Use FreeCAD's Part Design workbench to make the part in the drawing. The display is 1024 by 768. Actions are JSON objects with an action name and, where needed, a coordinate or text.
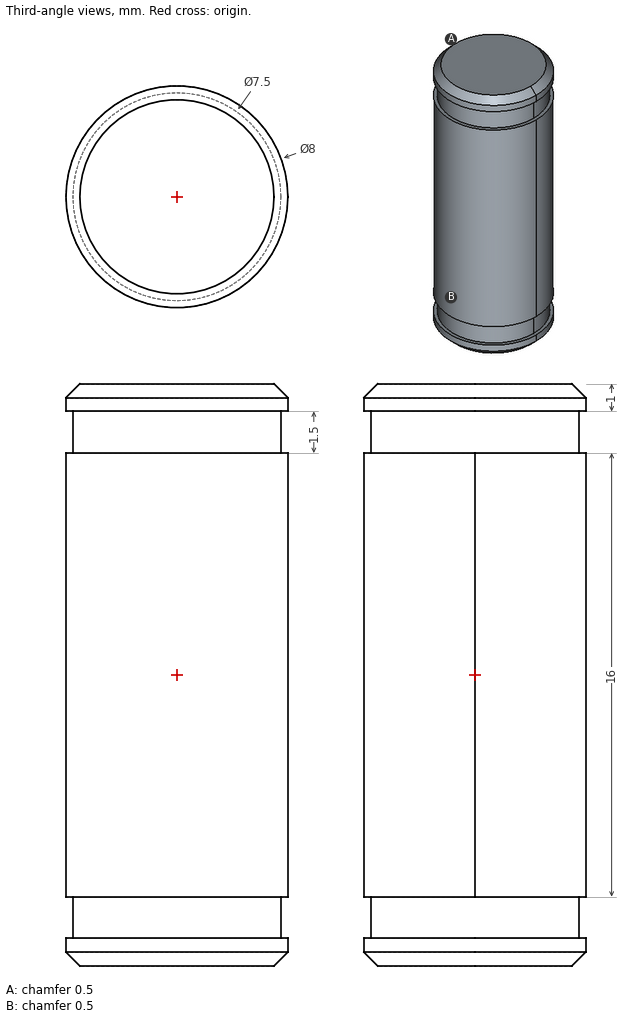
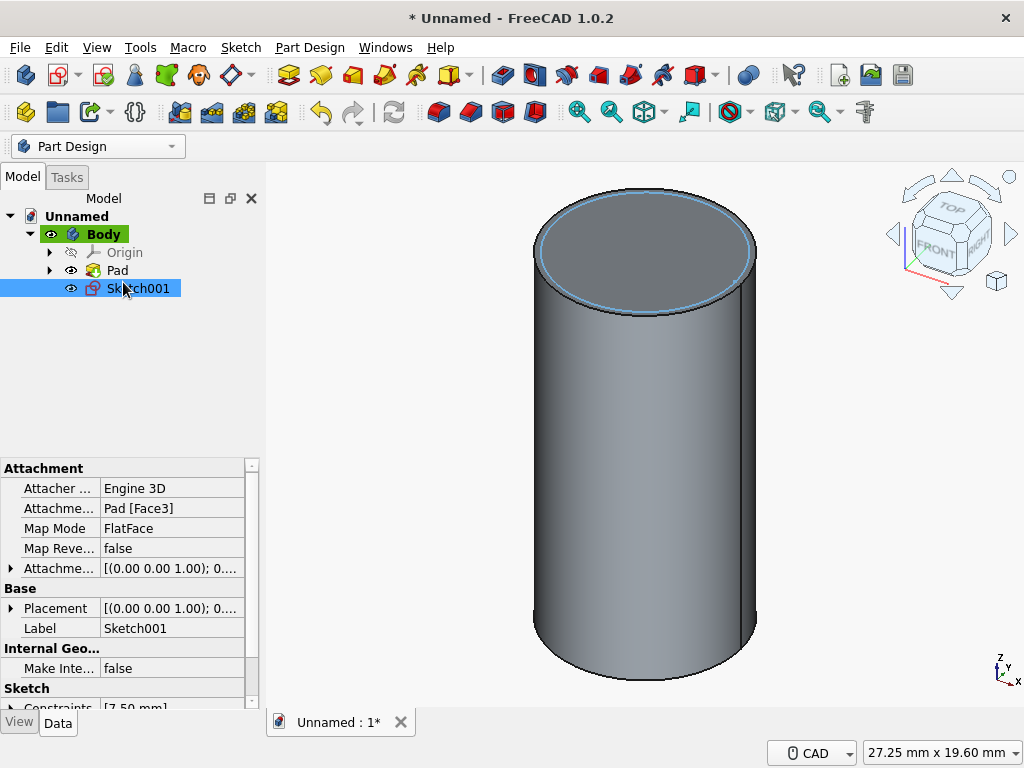
{"action": "left_click", "coordinate": [290, 76]}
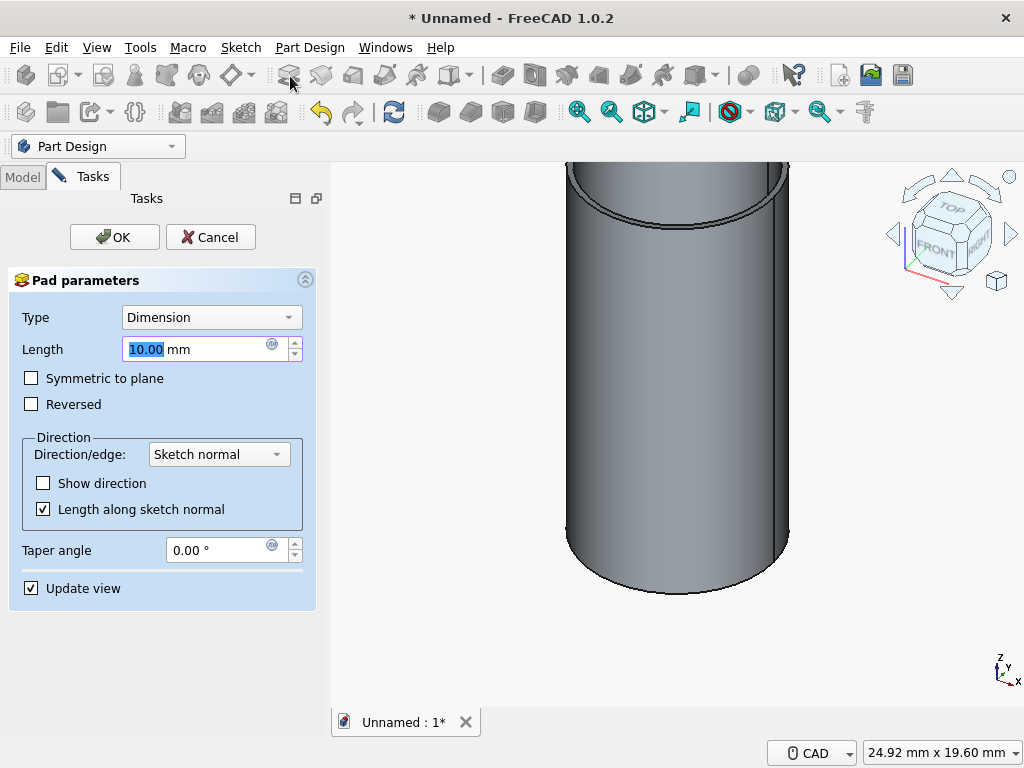
{"action": "type", "text": "1.5"}
{"action": "key", "text": "Tab"}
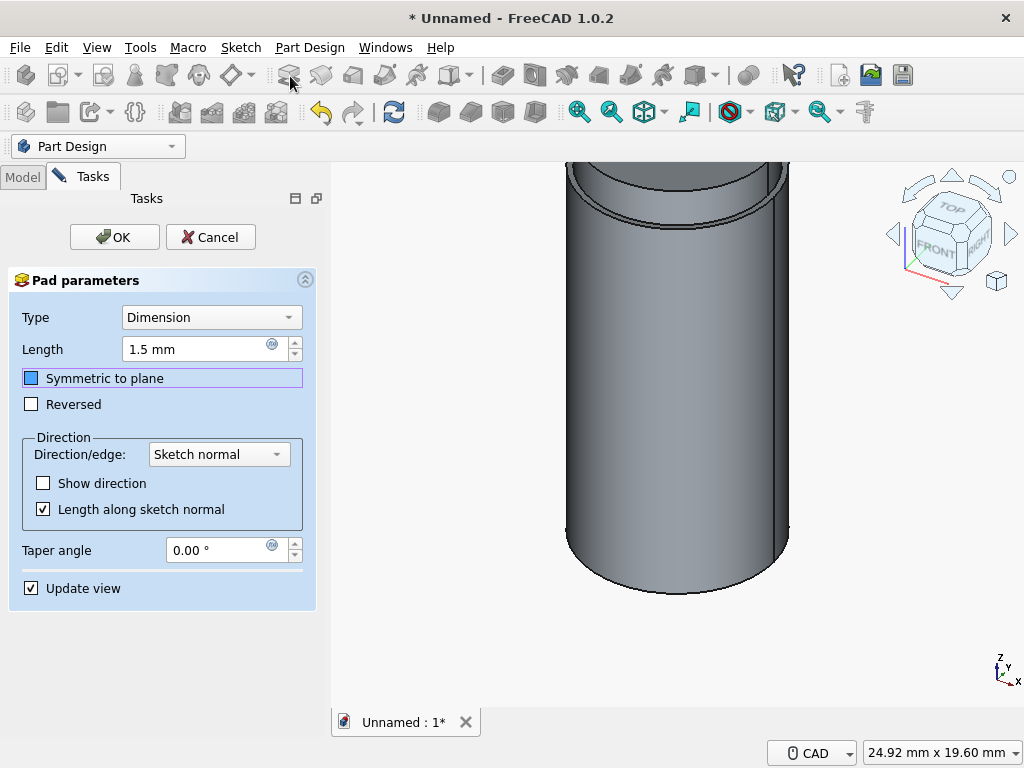
{"action": "left_click", "coordinate": [115, 237]}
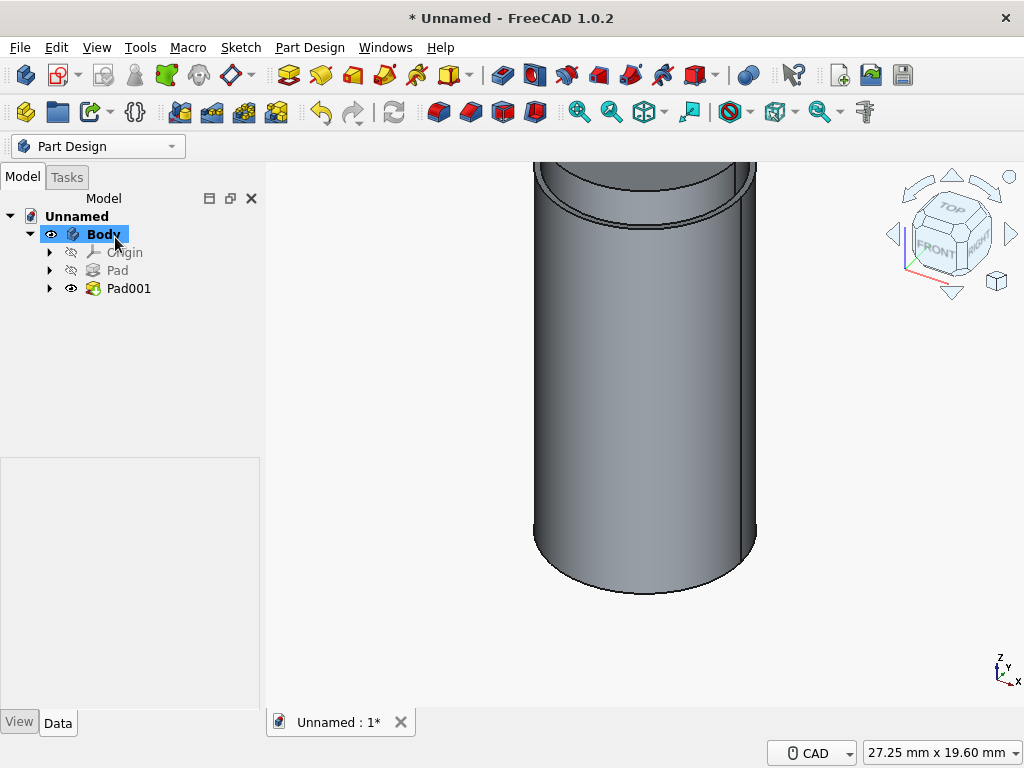
{"action": "key", "text": "v f"}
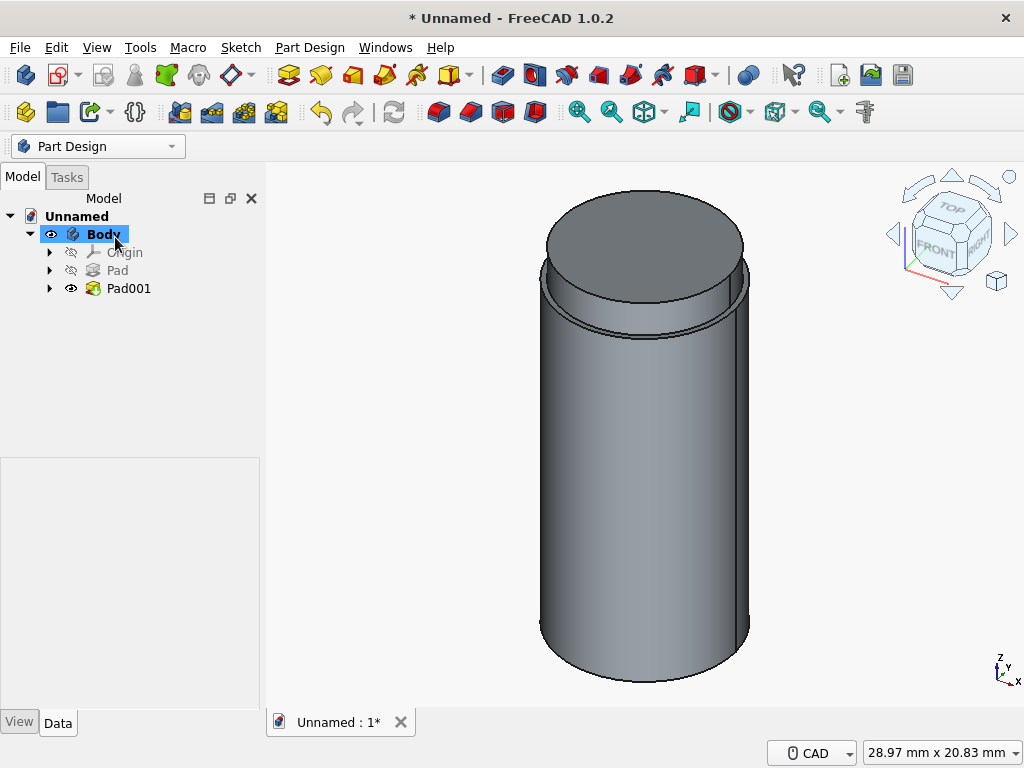
{"action": "left_click", "coordinate": [50, 252]}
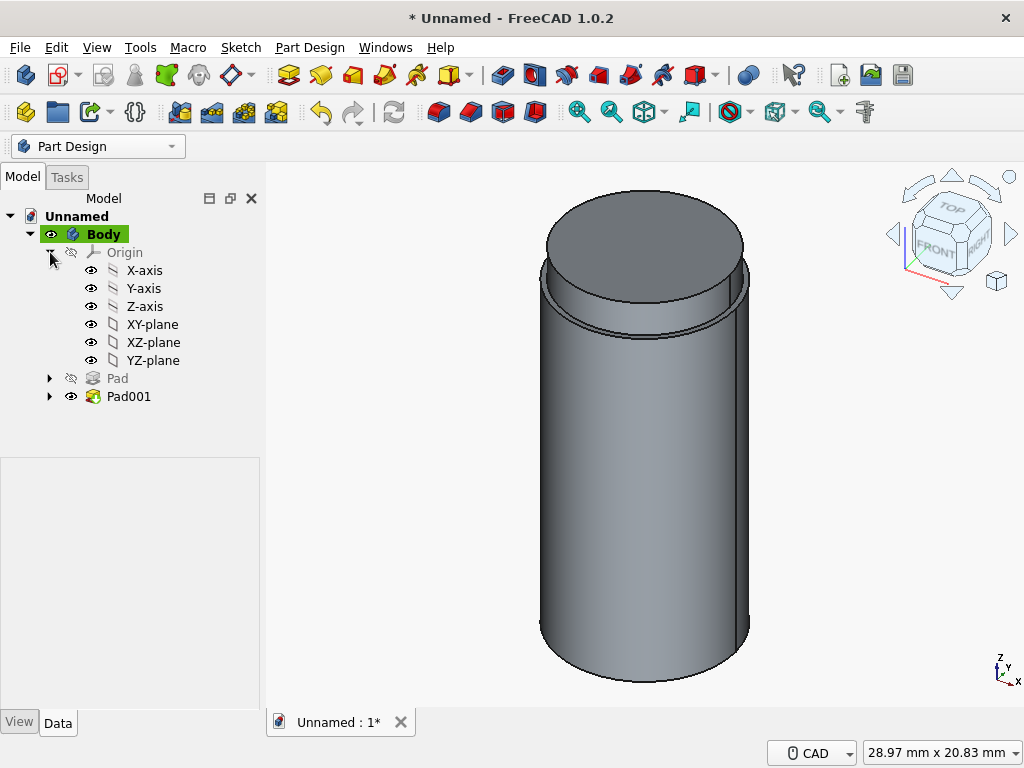
{"action": "left_click", "coordinate": [136, 324]}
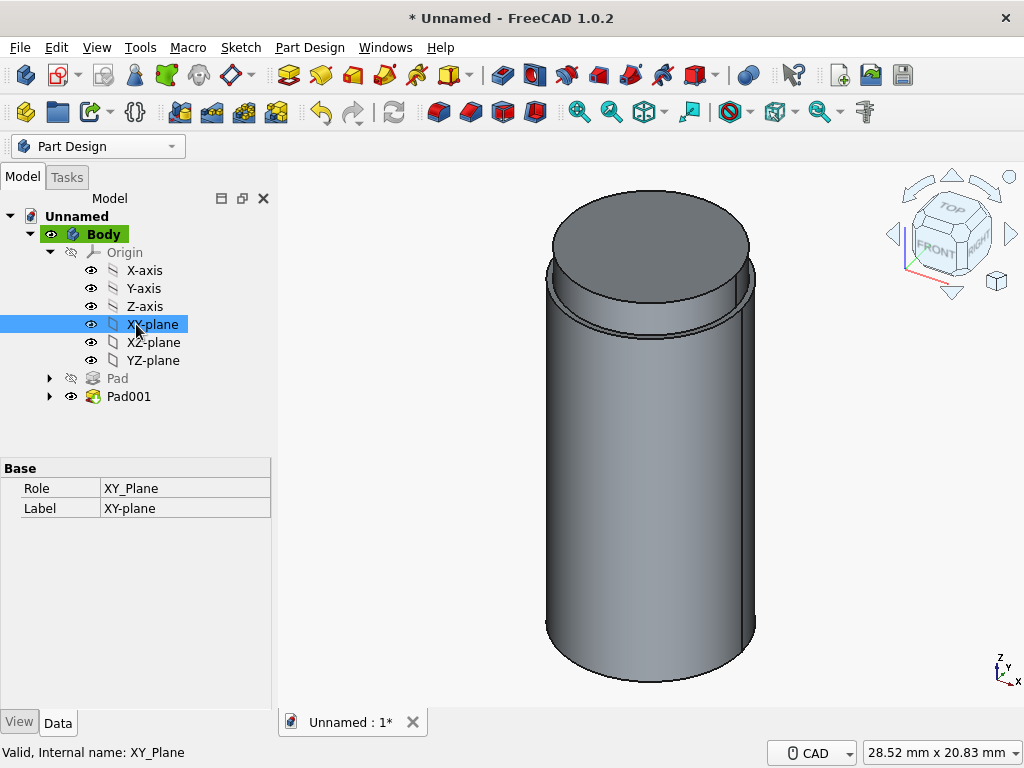
{"action": "left_click", "coordinate": [232, 76]}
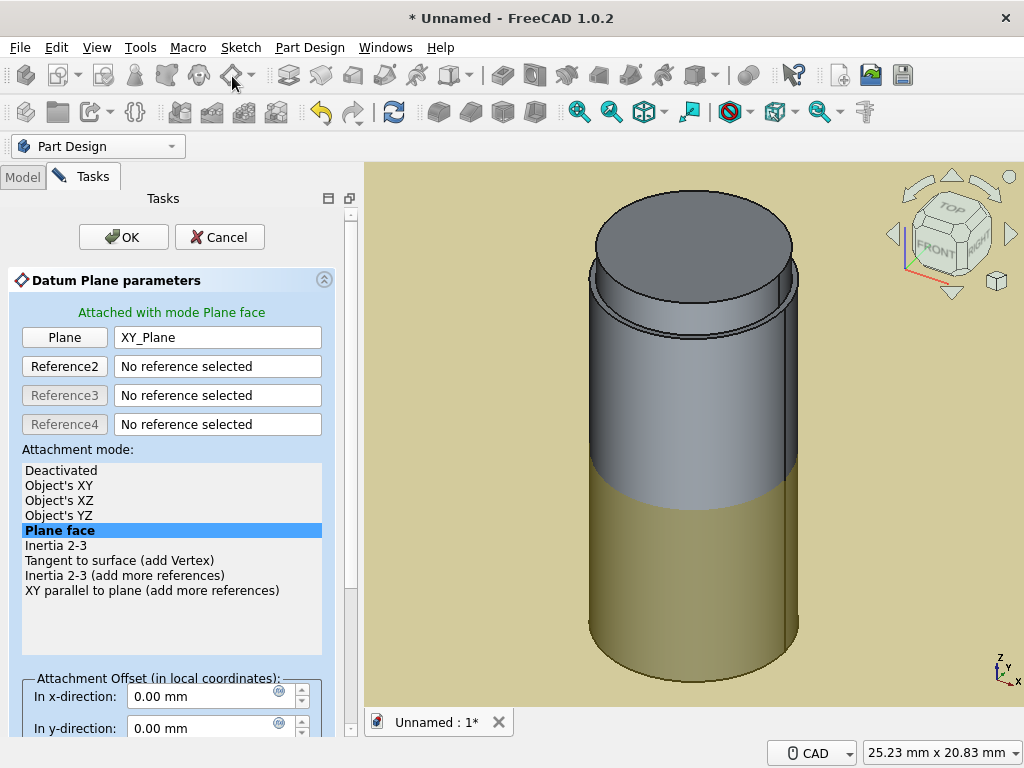
{"action": "scroll", "coordinate": [351, 472], "scroll_direction": "down", "scroll_amount": 2}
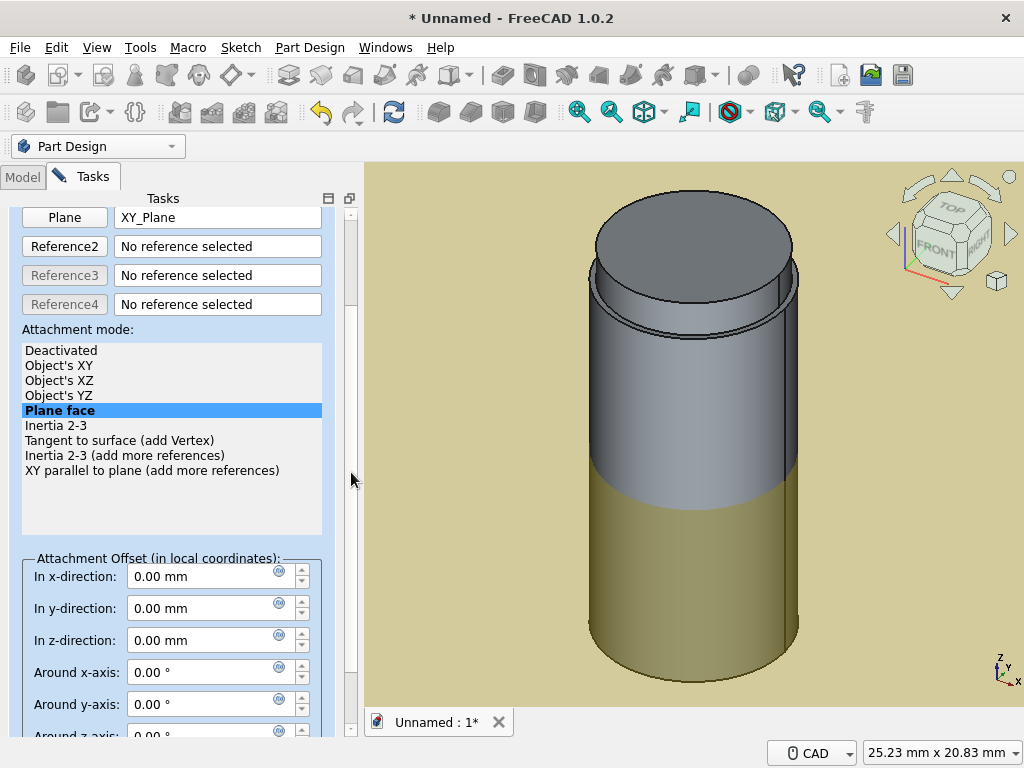
{"action": "triple_click", "coordinate": [210, 640]}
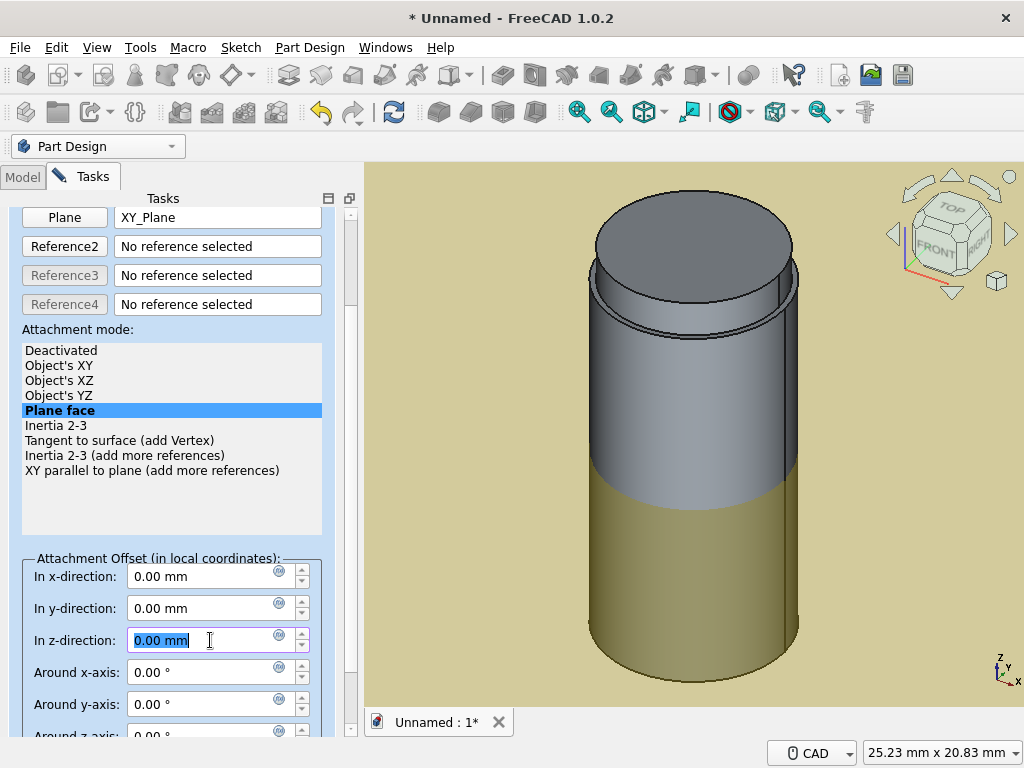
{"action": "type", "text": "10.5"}
{"action": "key", "text": "Tab"}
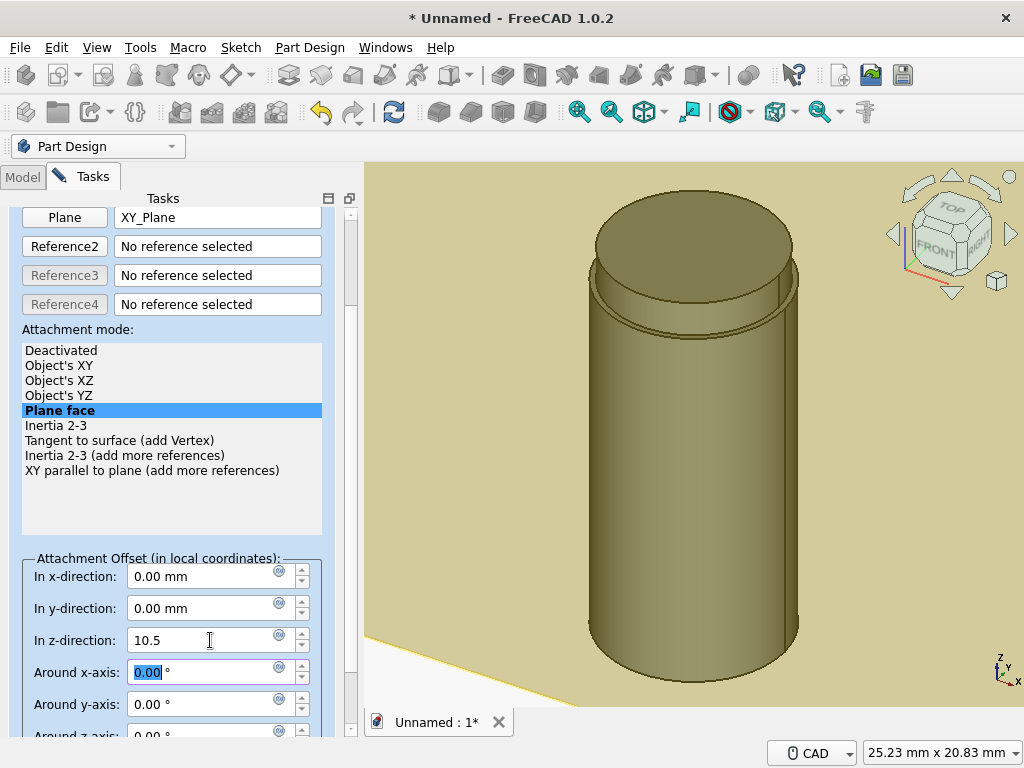
{"action": "scroll", "coordinate": [351, 472], "scroll_direction": "up", "scroll_amount": 3}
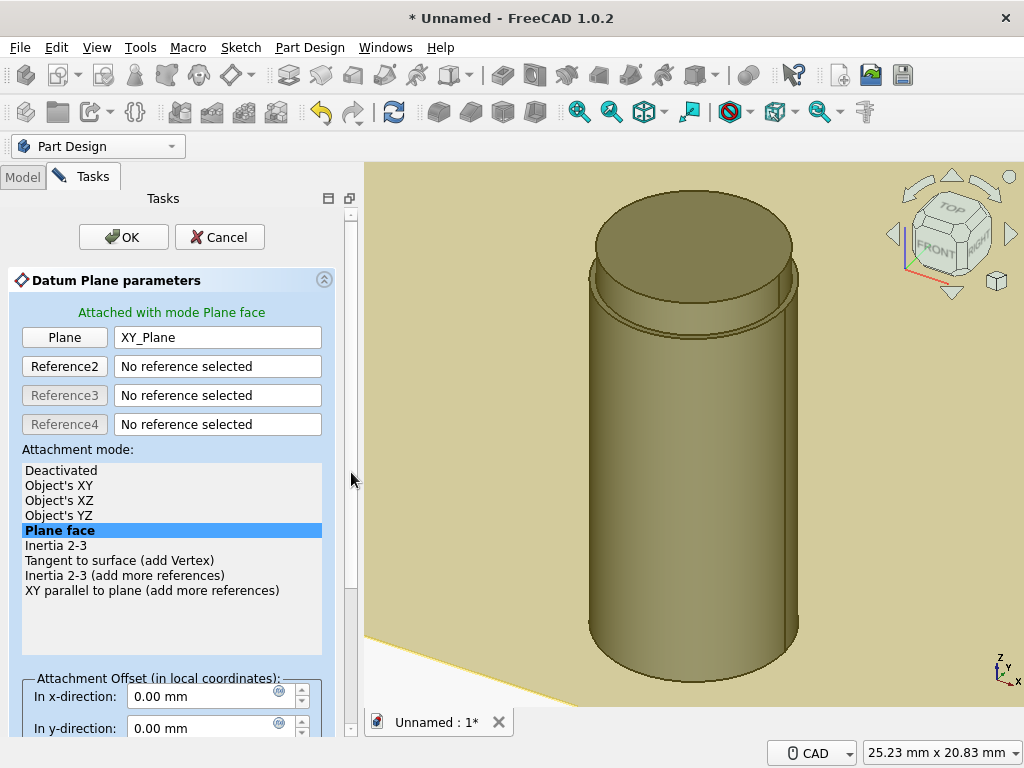
{"action": "left_click", "coordinate": [124, 237]}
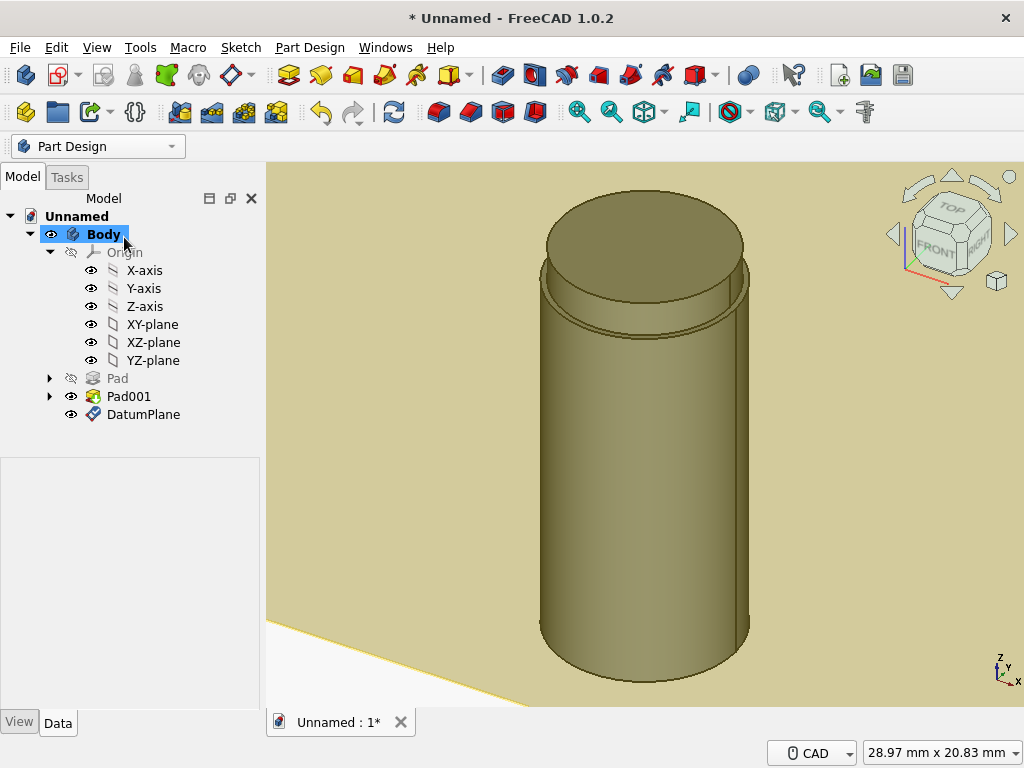
{"action": "left_click", "coordinate": [116, 414]}